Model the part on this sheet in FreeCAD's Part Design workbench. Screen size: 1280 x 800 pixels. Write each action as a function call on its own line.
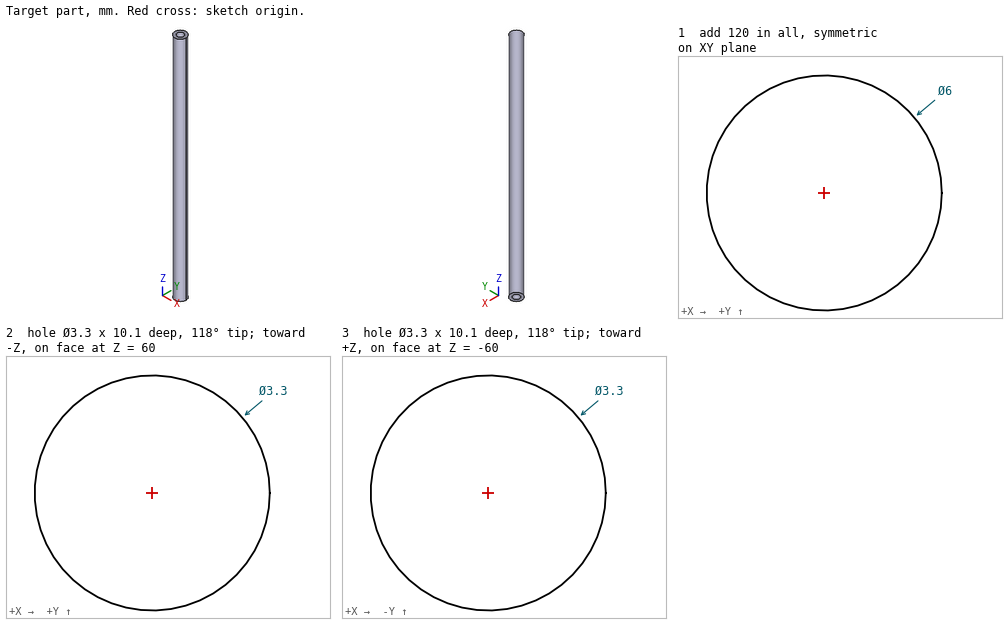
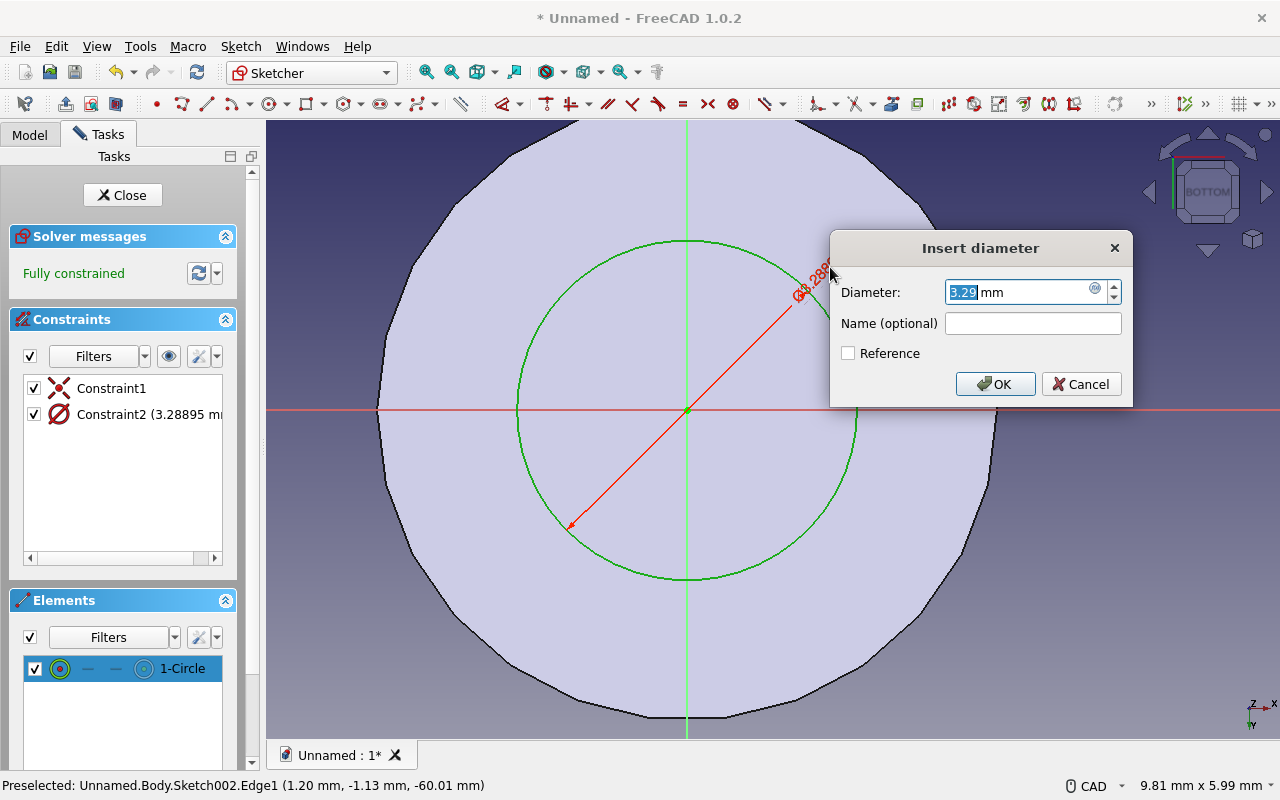
text(3.3)
key(Return)
key(Escape)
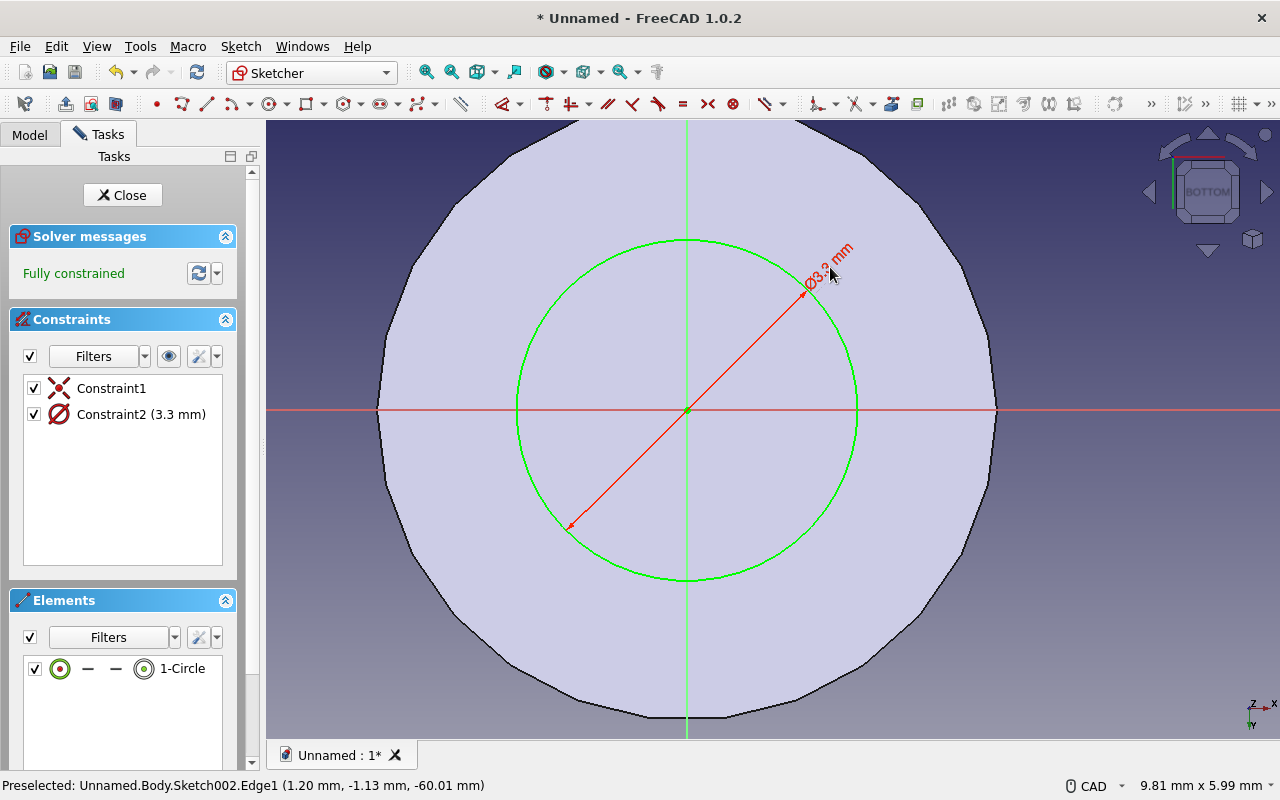
click(123, 195)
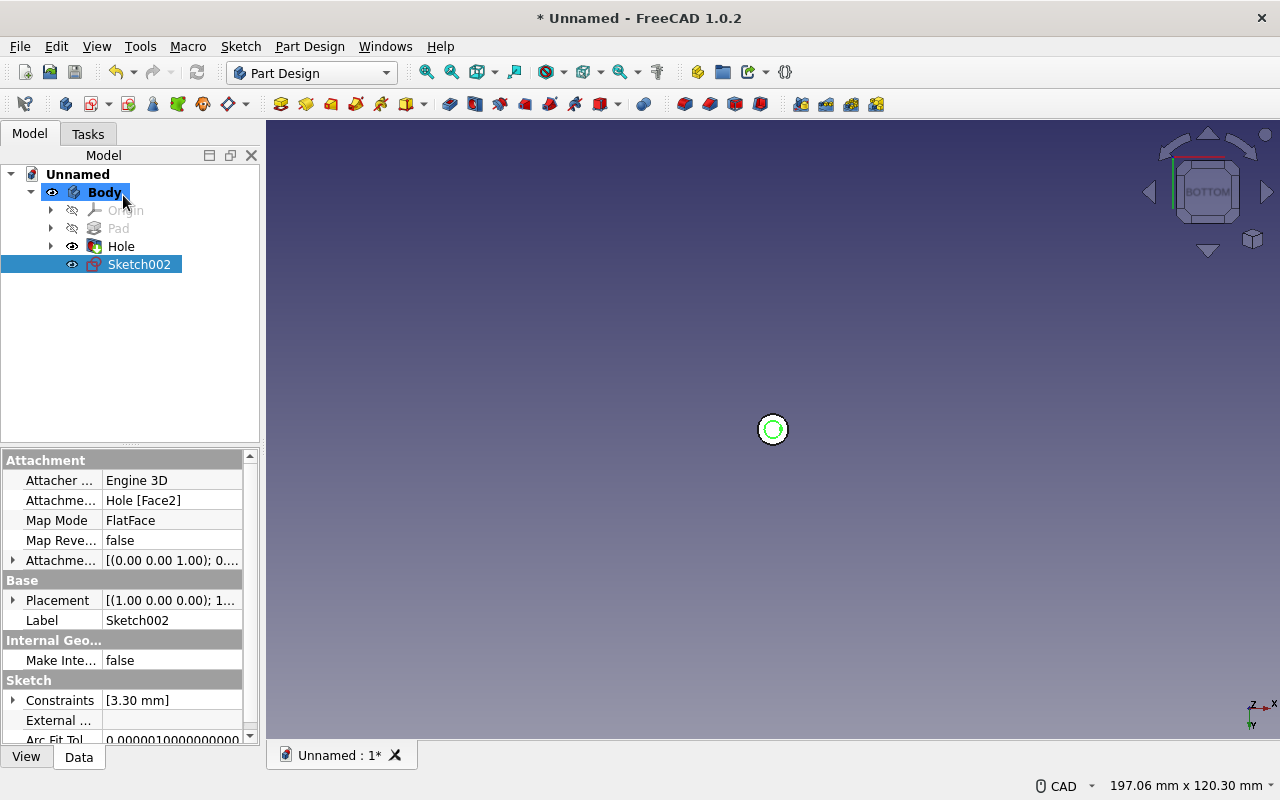
click(475, 104)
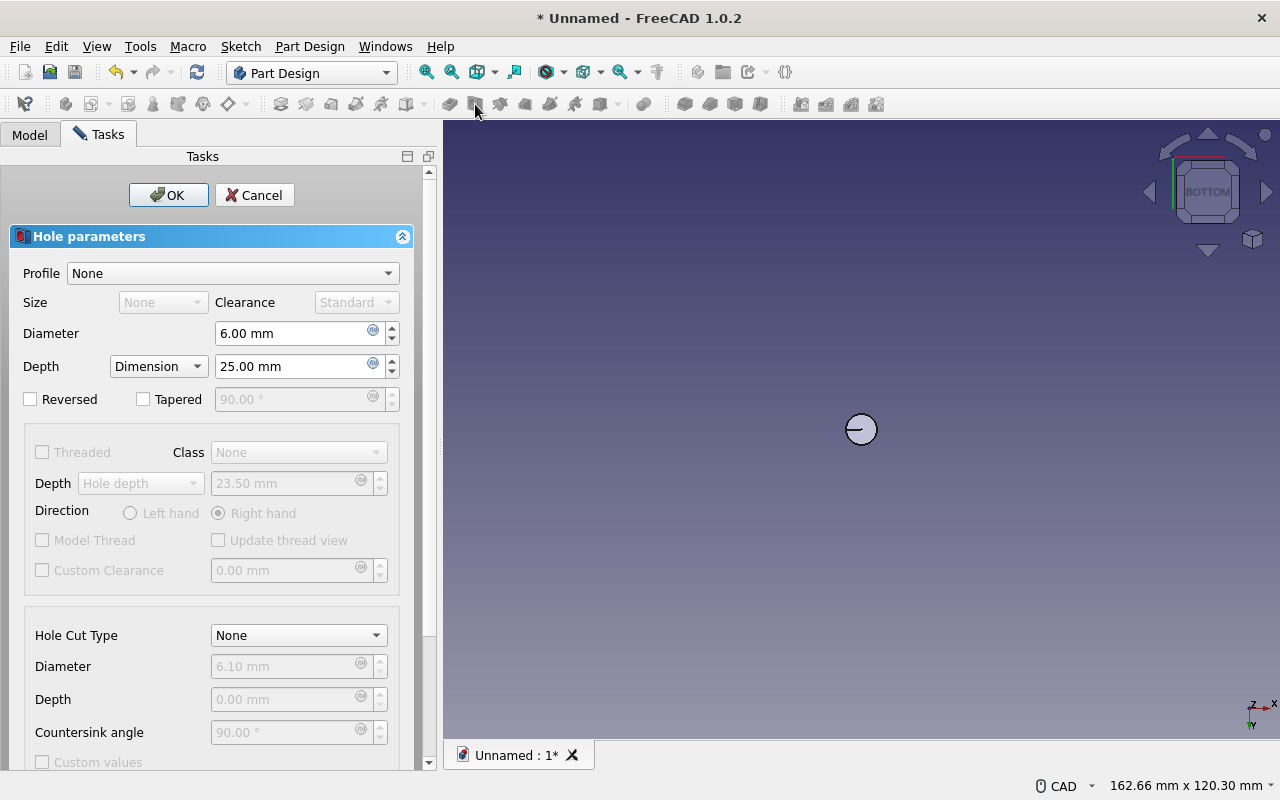
triple_click(300, 334)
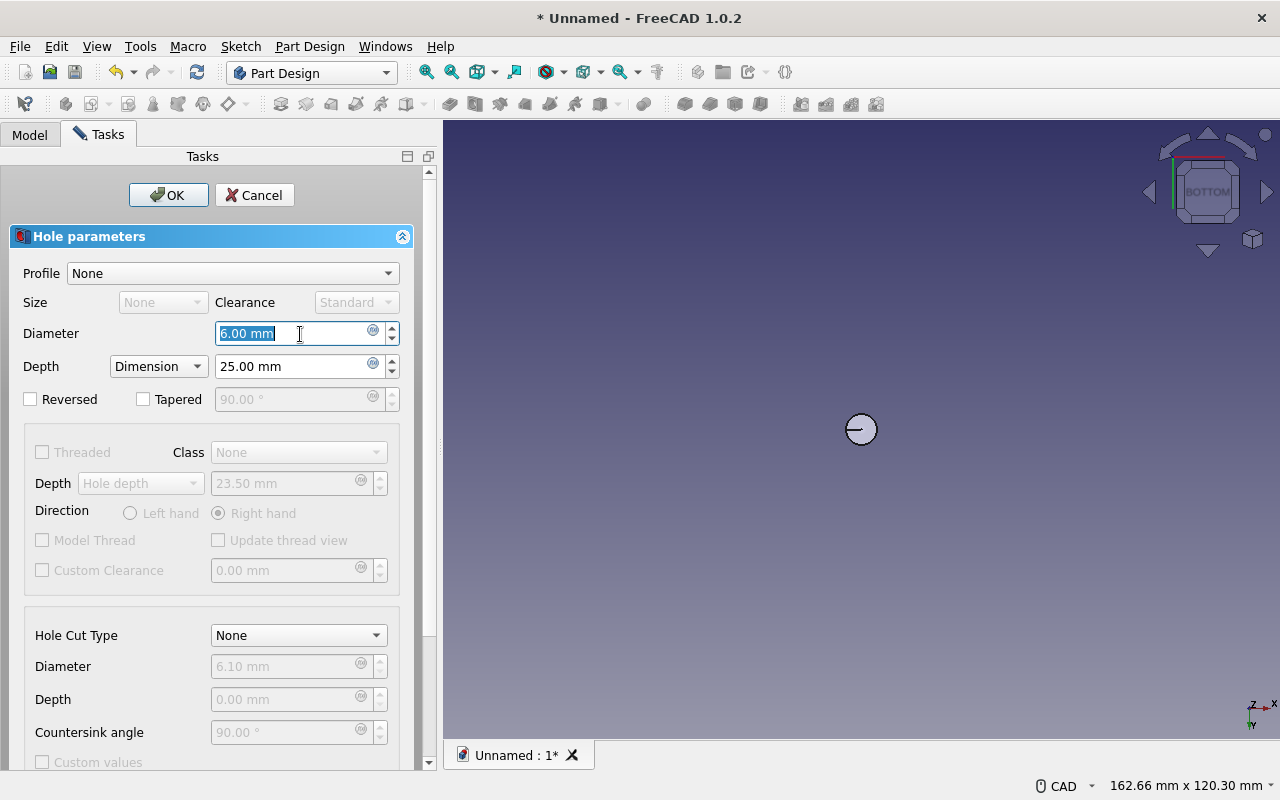
text(3.3)
key(Tab)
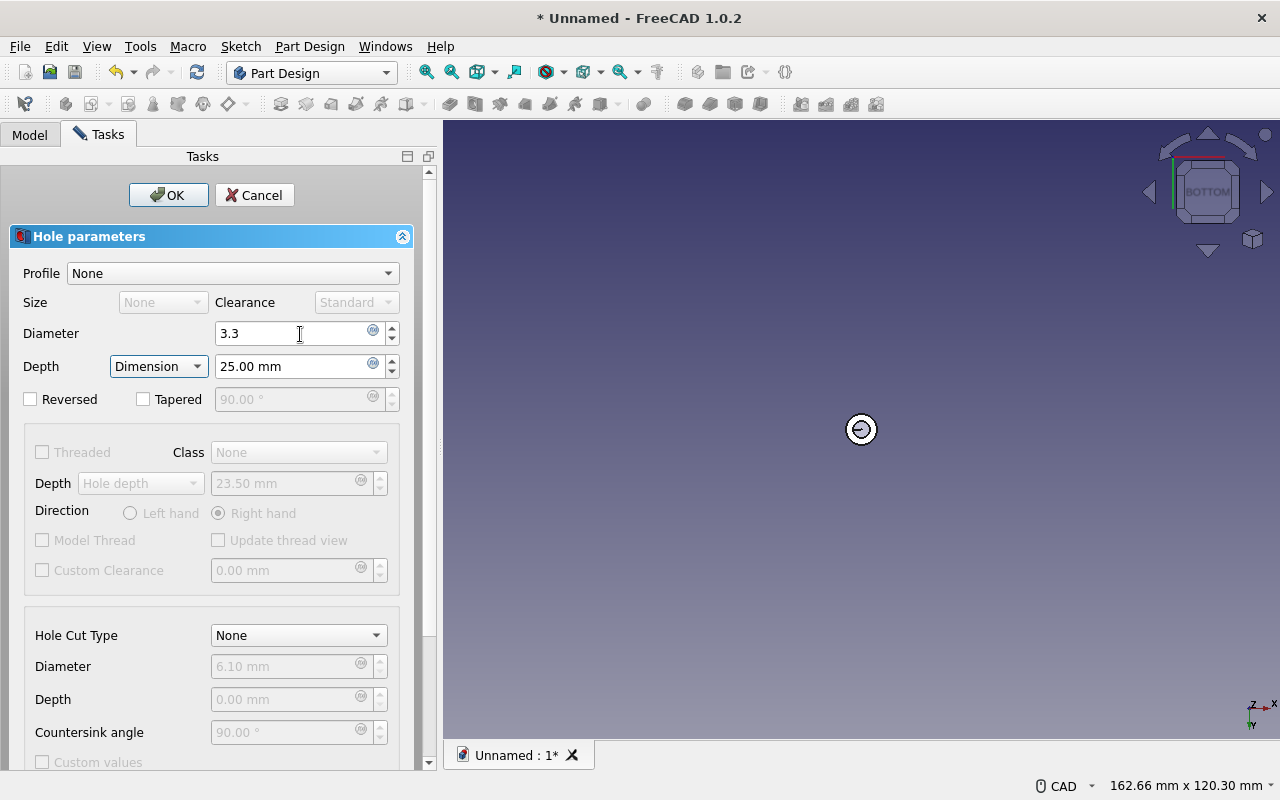
triple_click(300, 366)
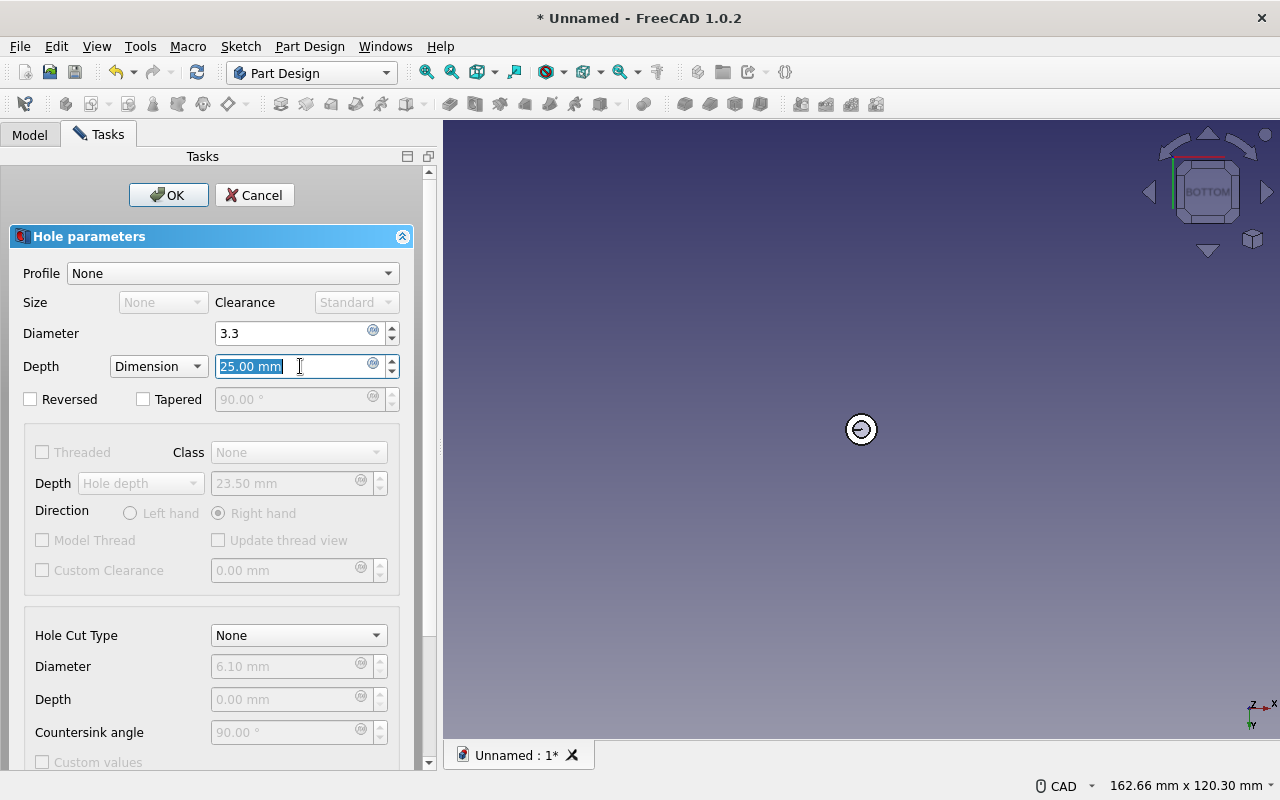
text(10.1)
key(Tab)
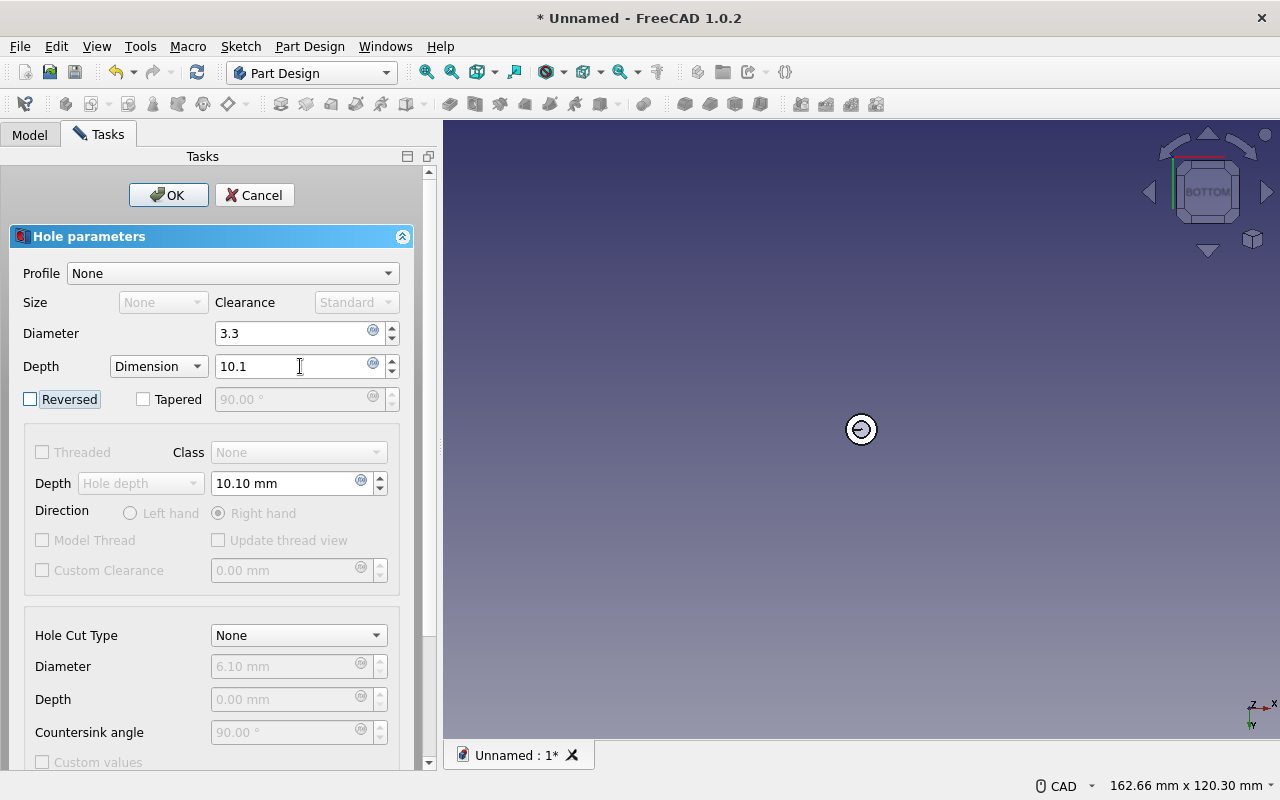
click(169, 195)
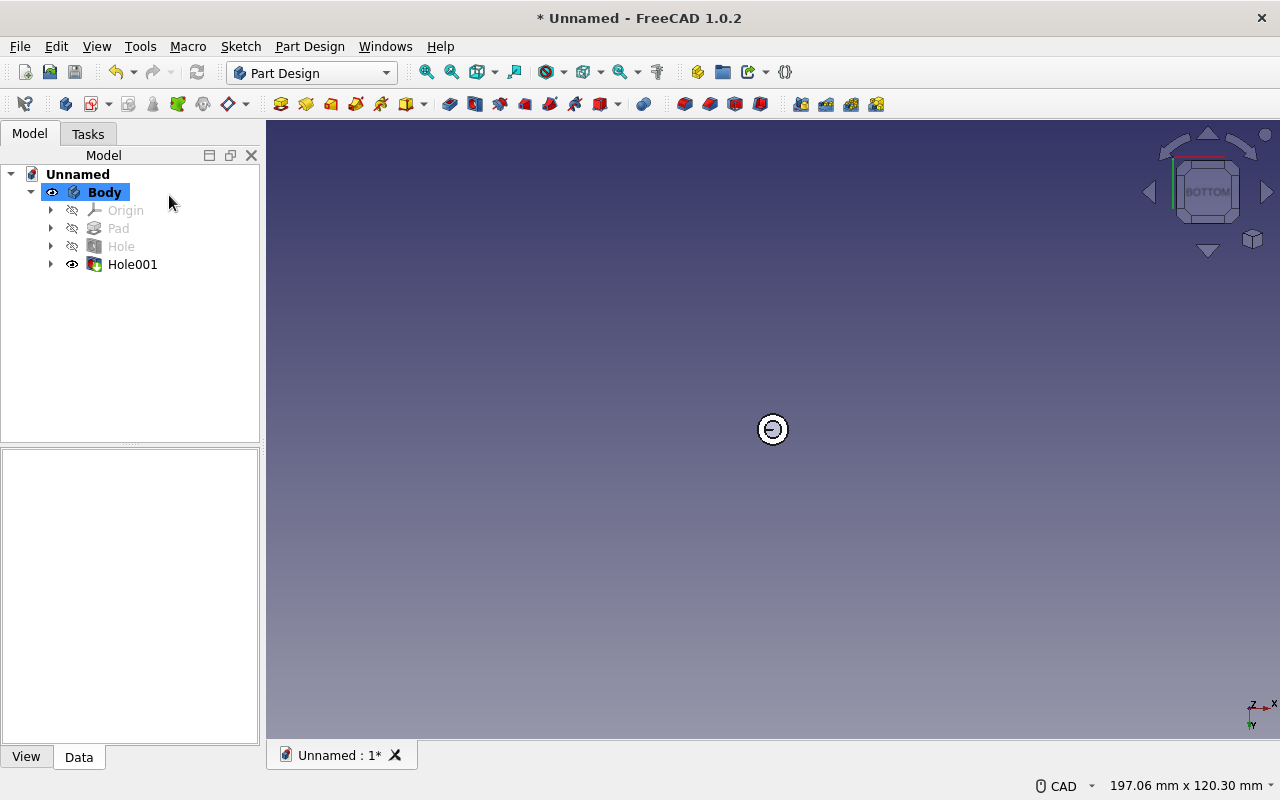
key(0)